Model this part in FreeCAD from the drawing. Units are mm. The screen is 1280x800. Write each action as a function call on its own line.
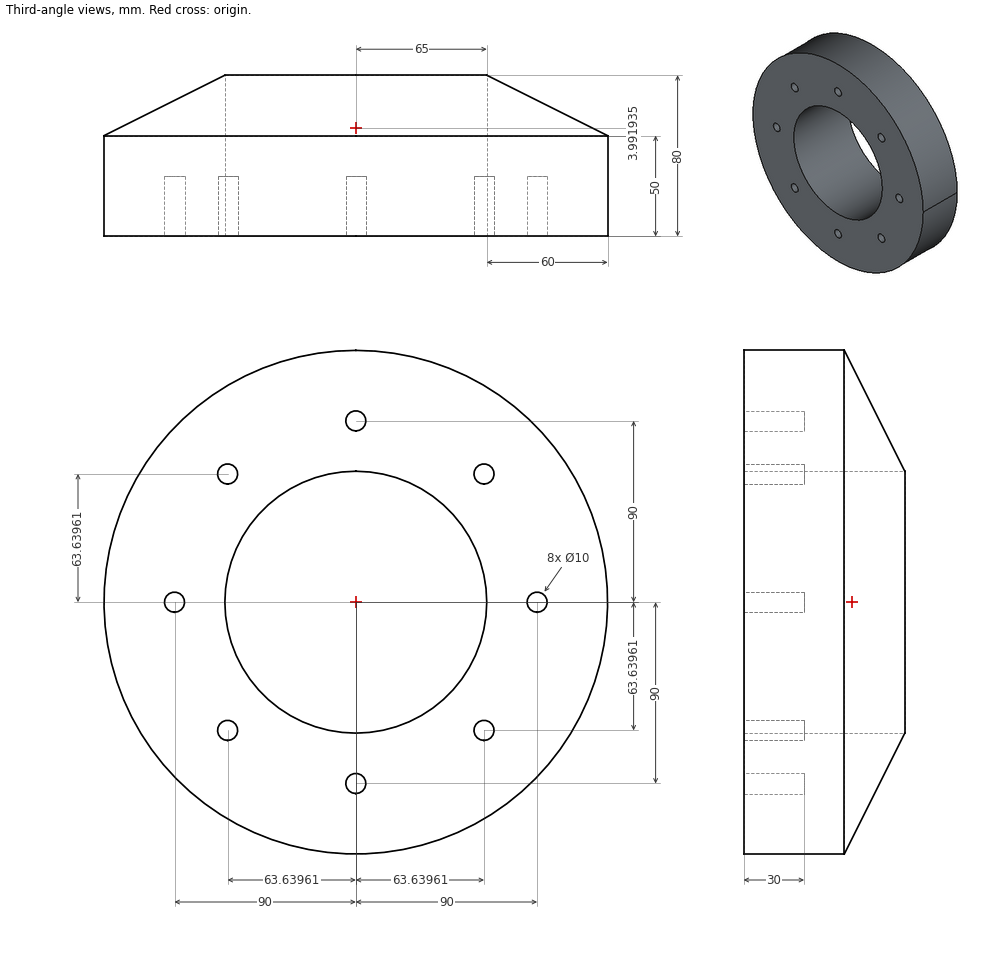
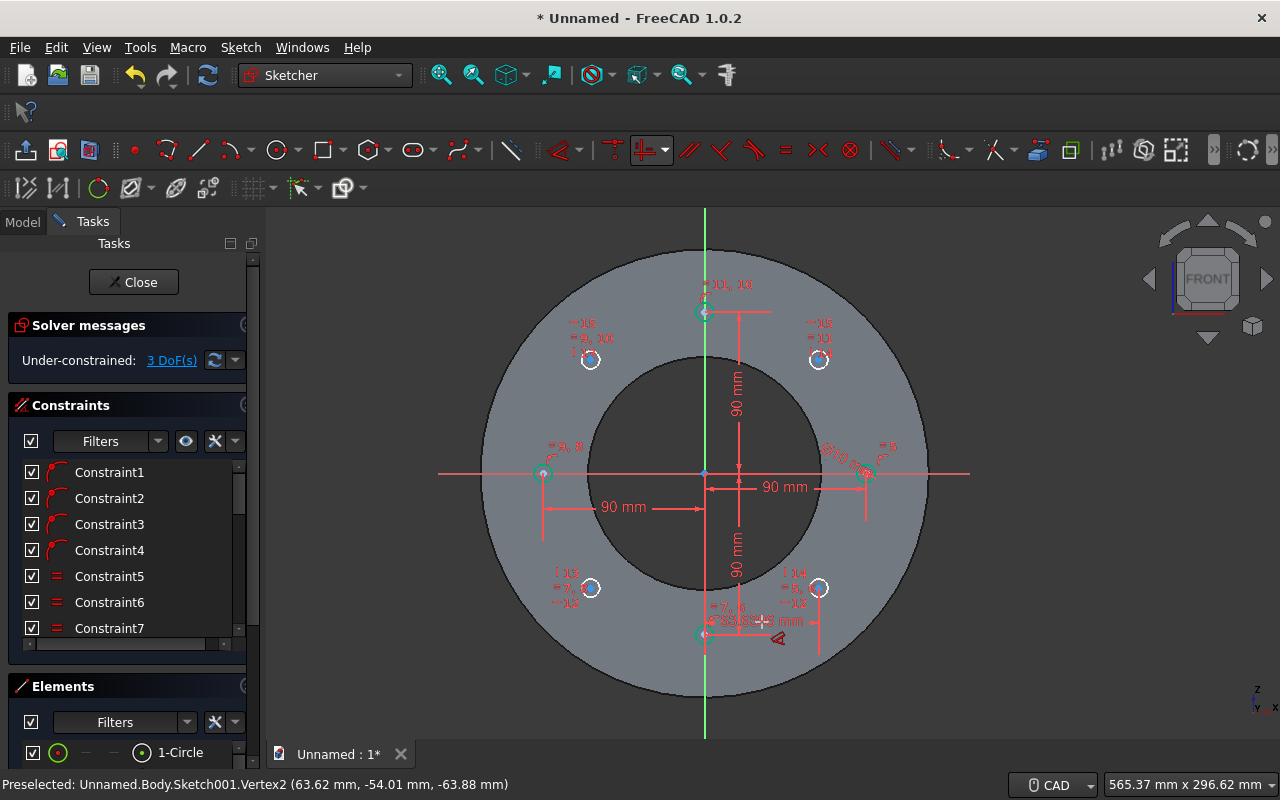
click(819, 588)
click(853, 531)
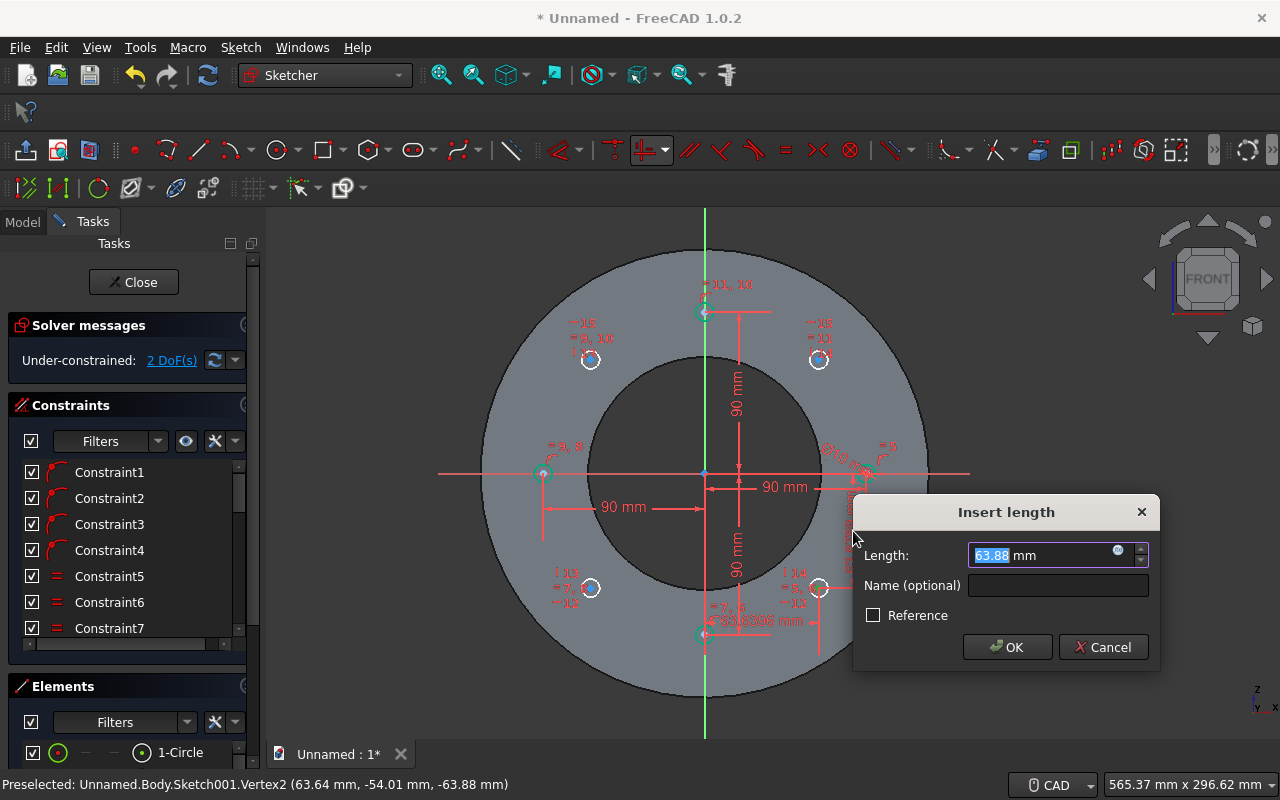
text(63.63961)
key(Return)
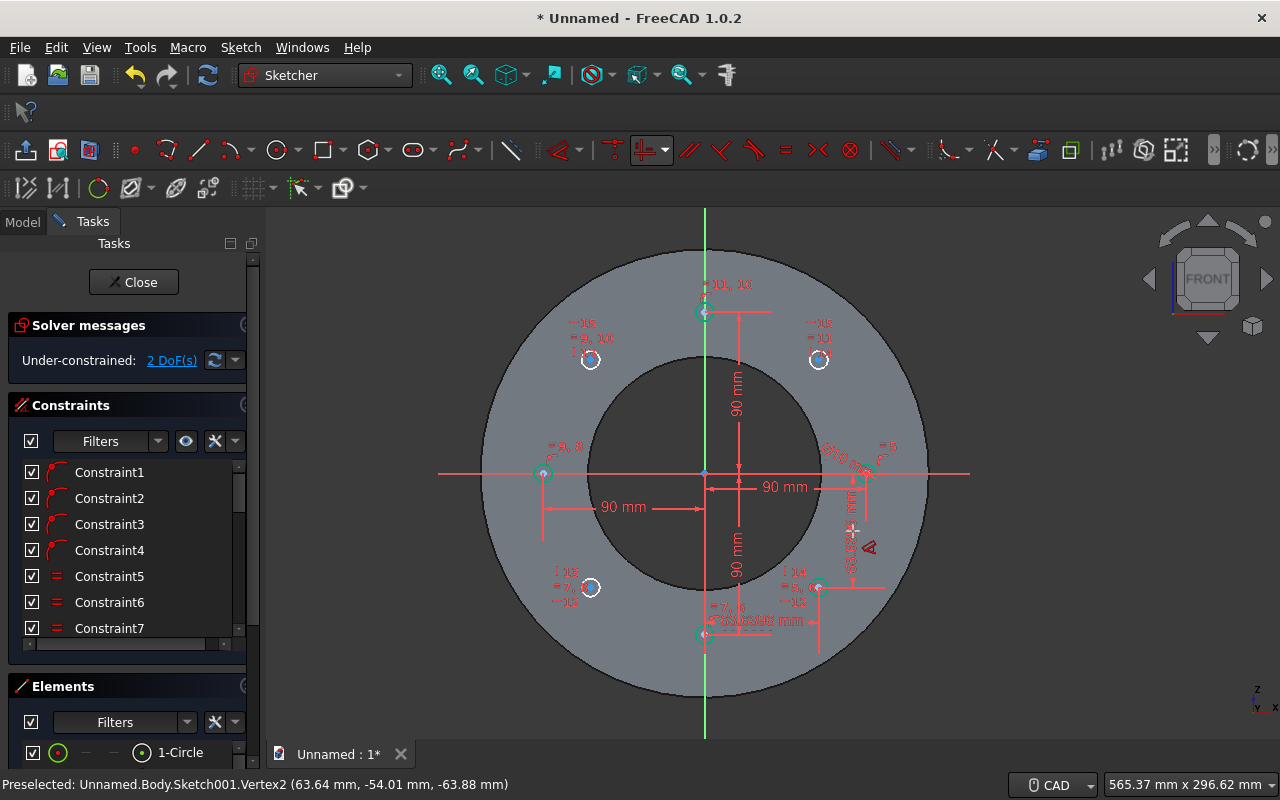
click(591, 588)
click(648, 622)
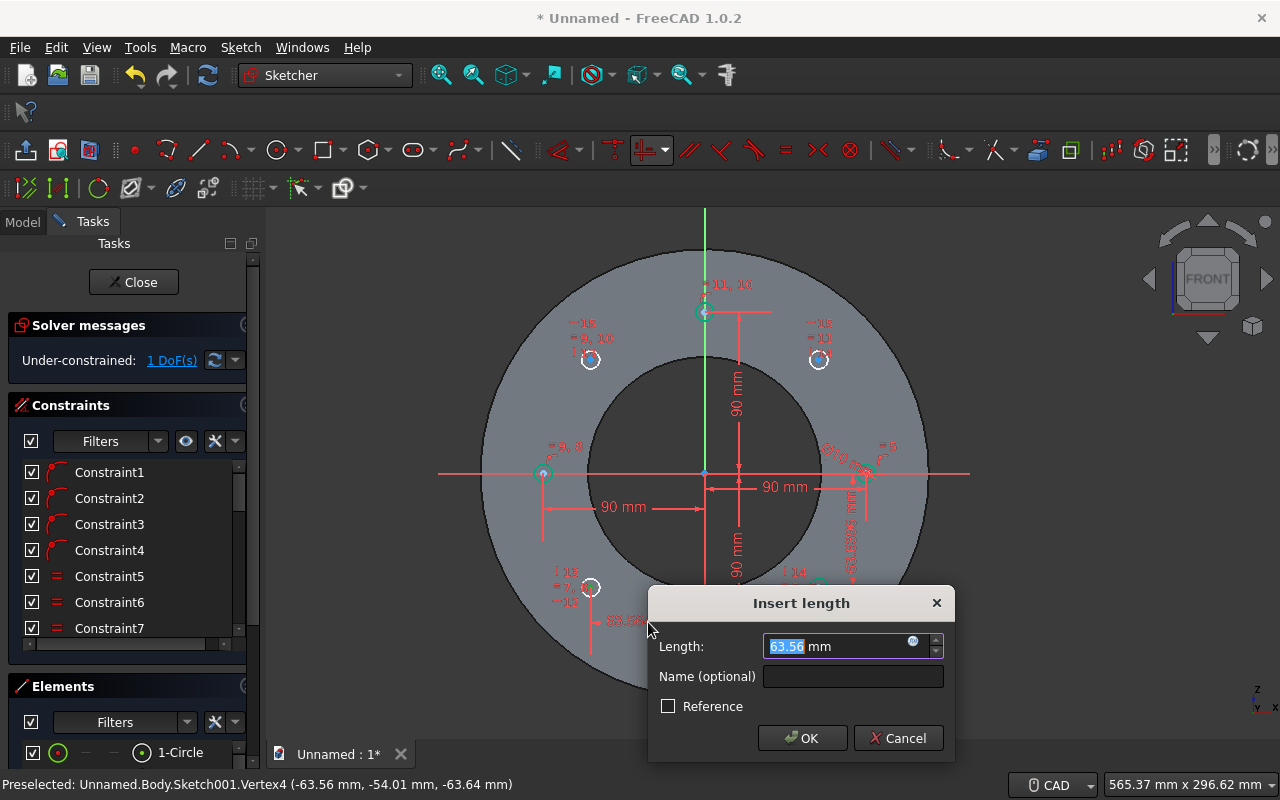
text(63.63961)
key(Return)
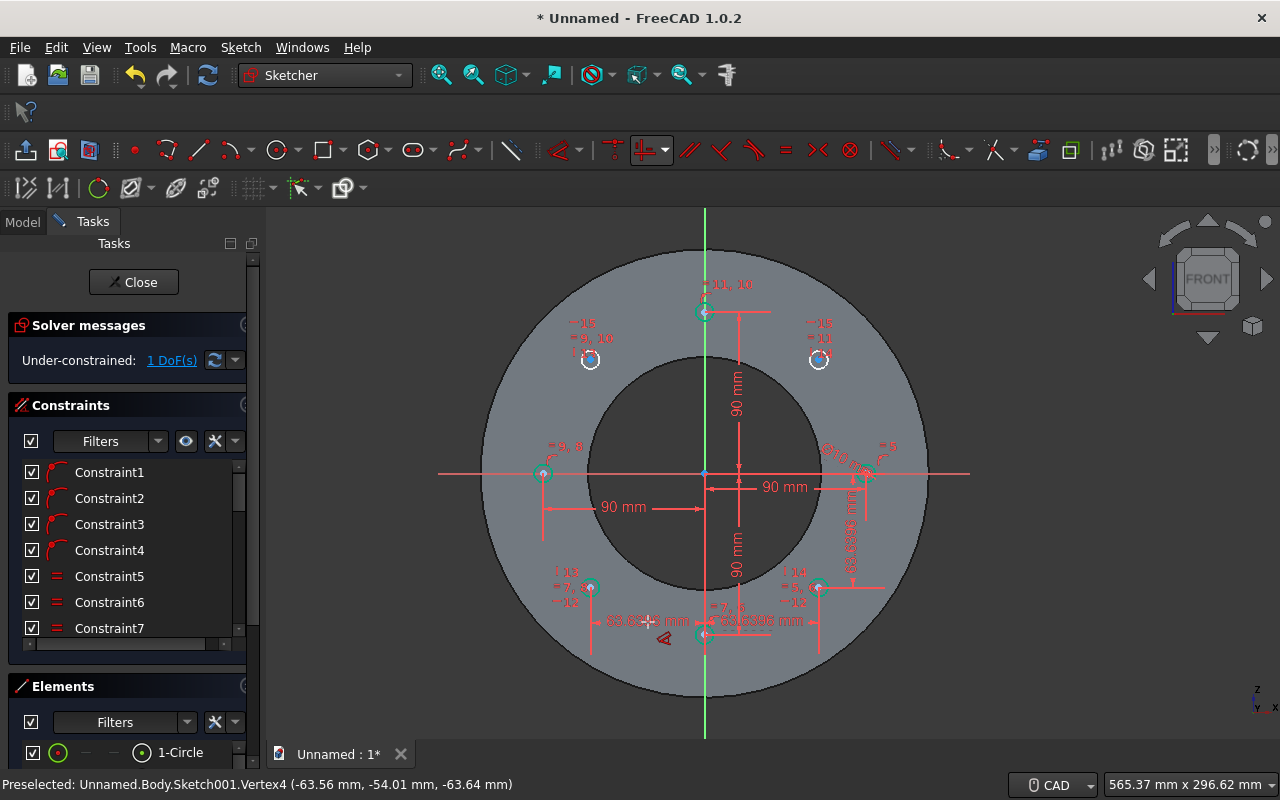
click(591, 360)
click(557, 417)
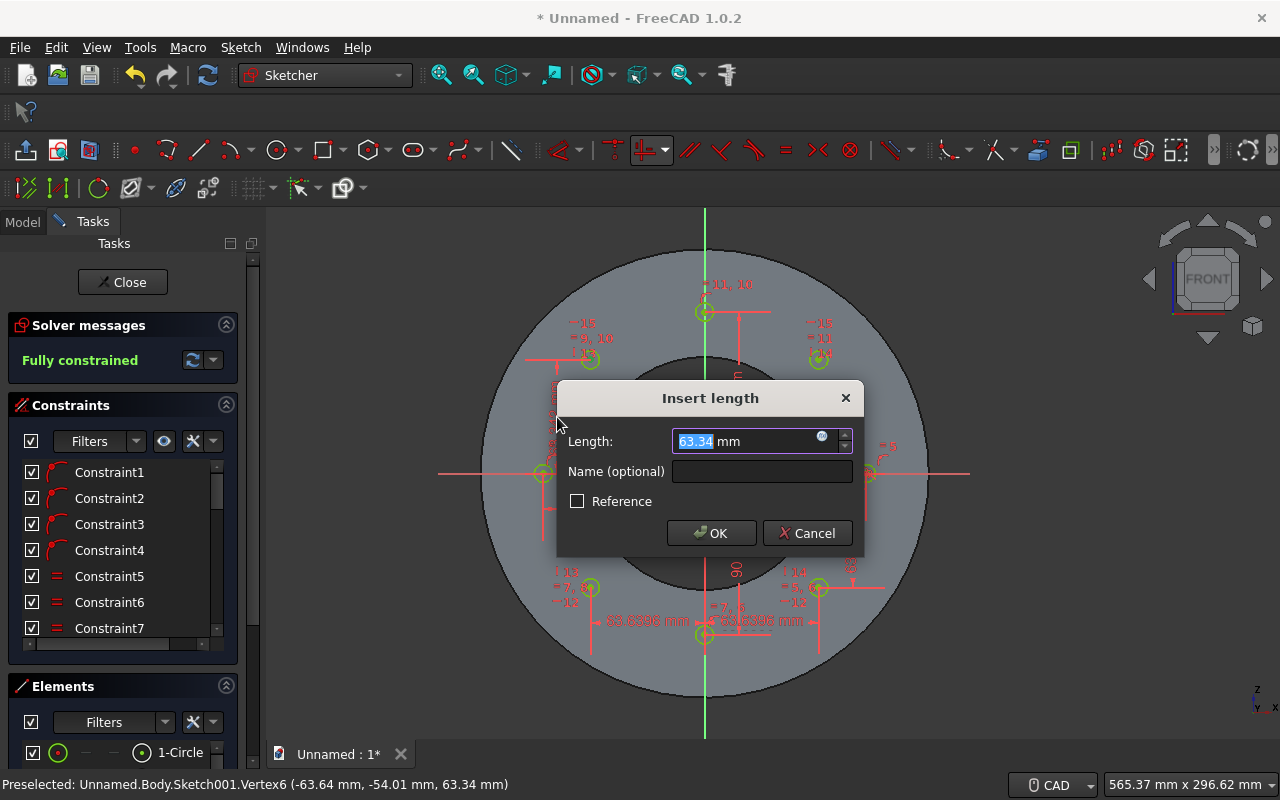
text(63.63961)
key(Return)
key(Escape)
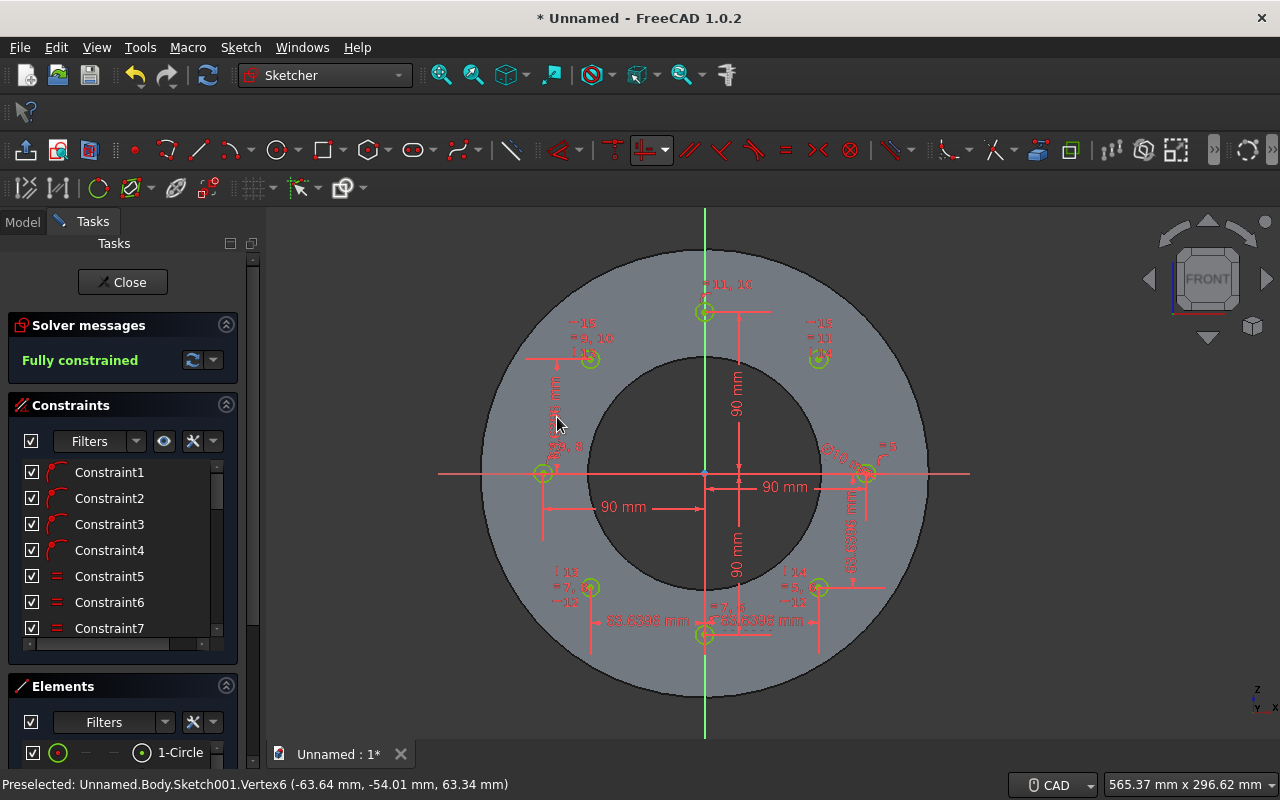
click(123, 282)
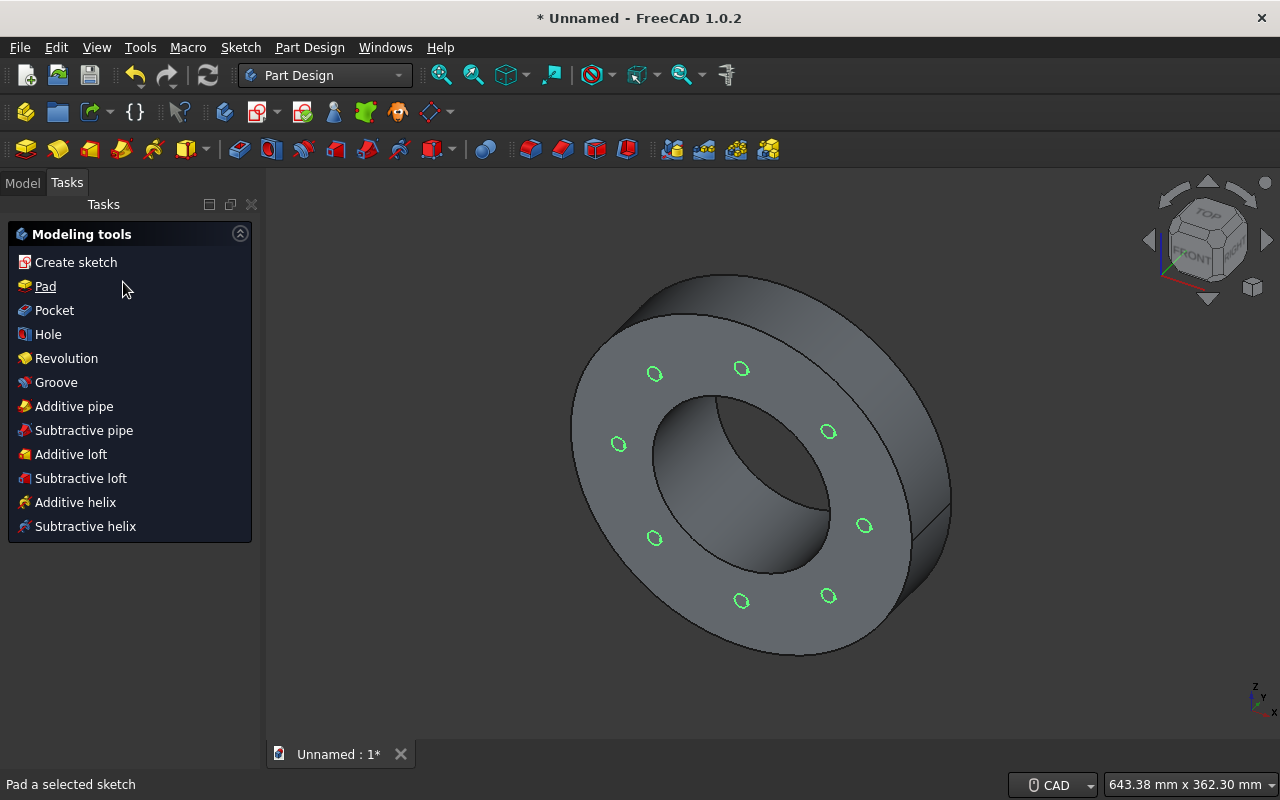
click(240, 150)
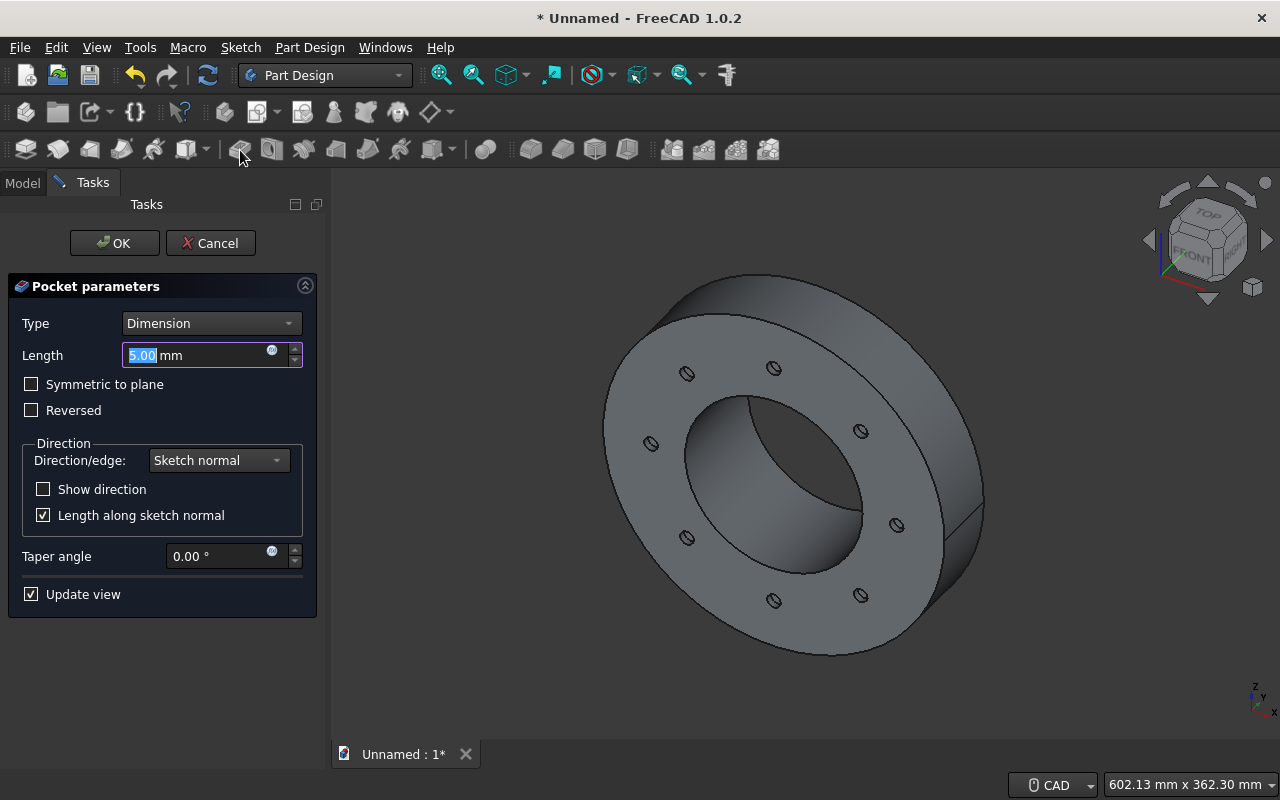
text(30)
key(Tab)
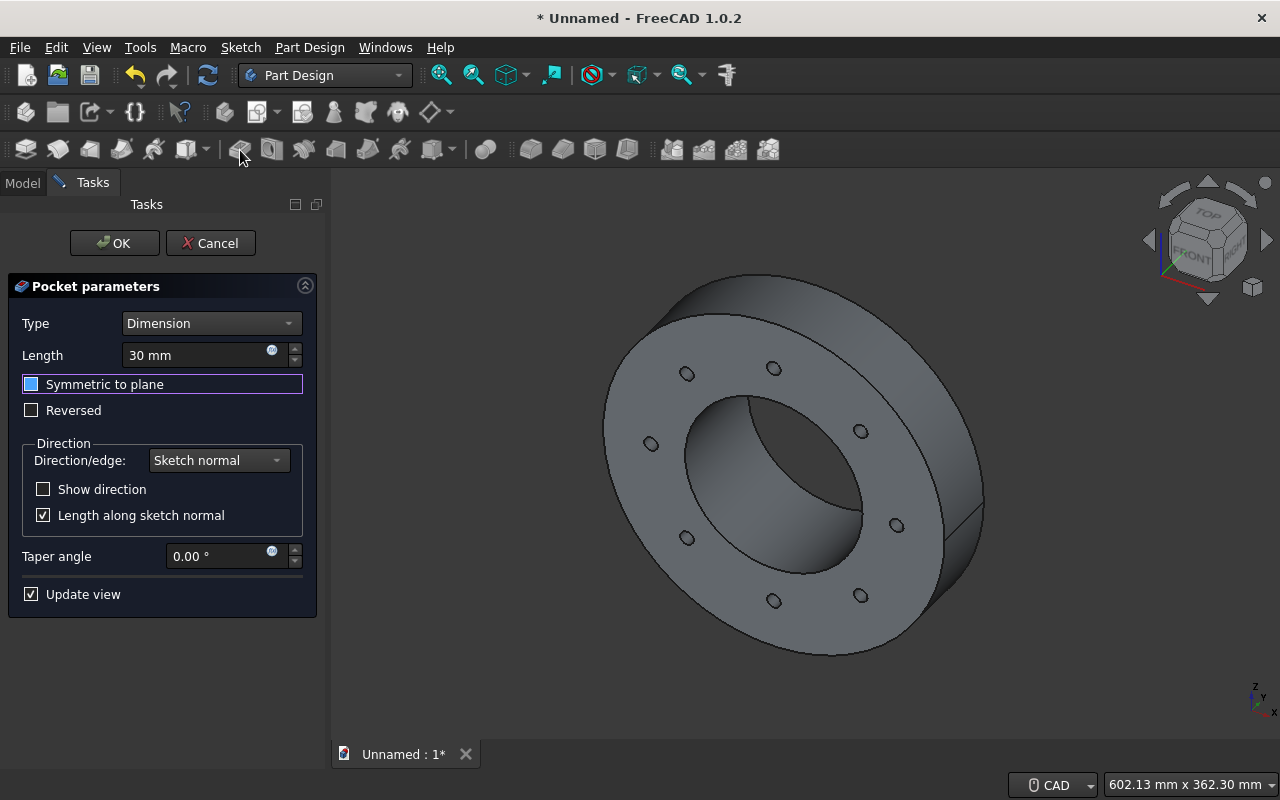
click(115, 243)